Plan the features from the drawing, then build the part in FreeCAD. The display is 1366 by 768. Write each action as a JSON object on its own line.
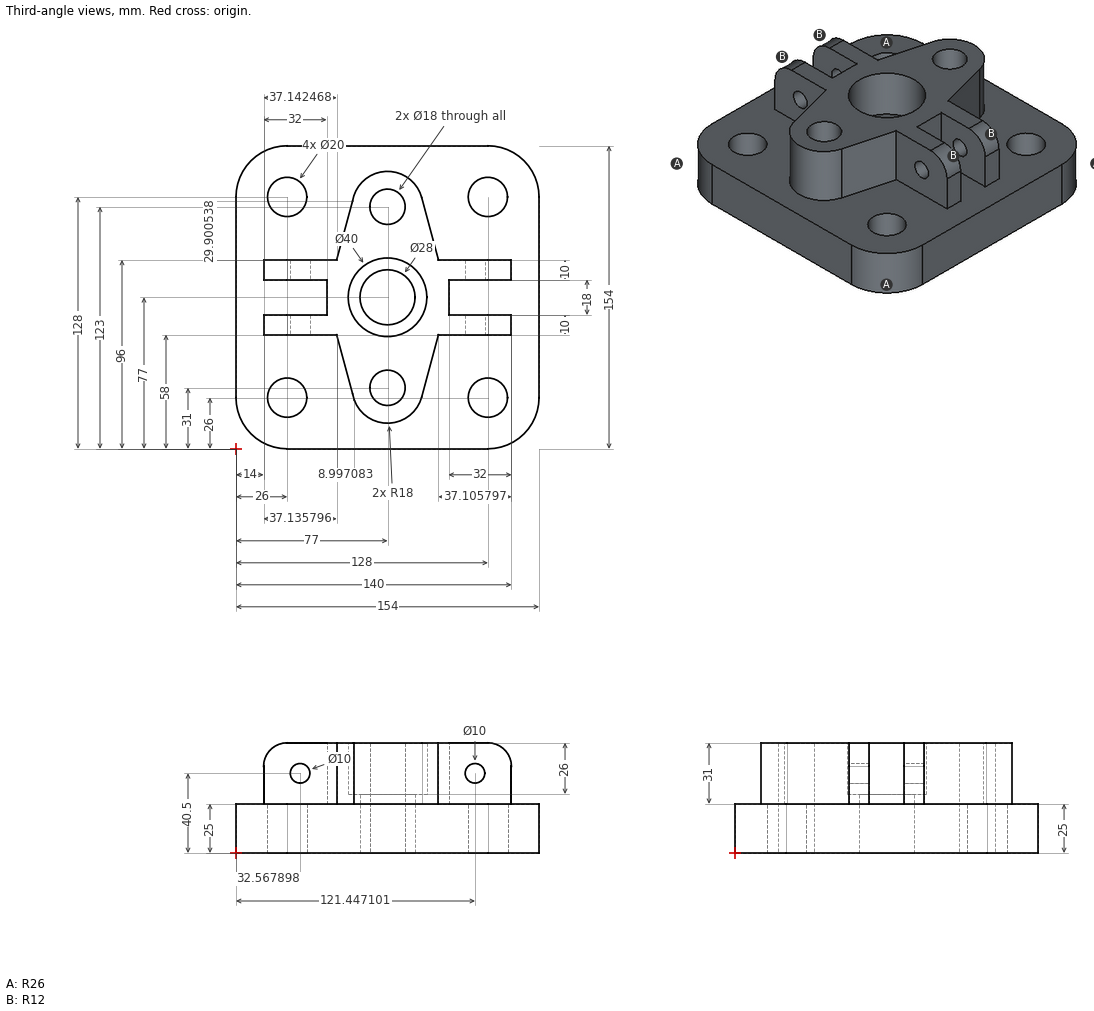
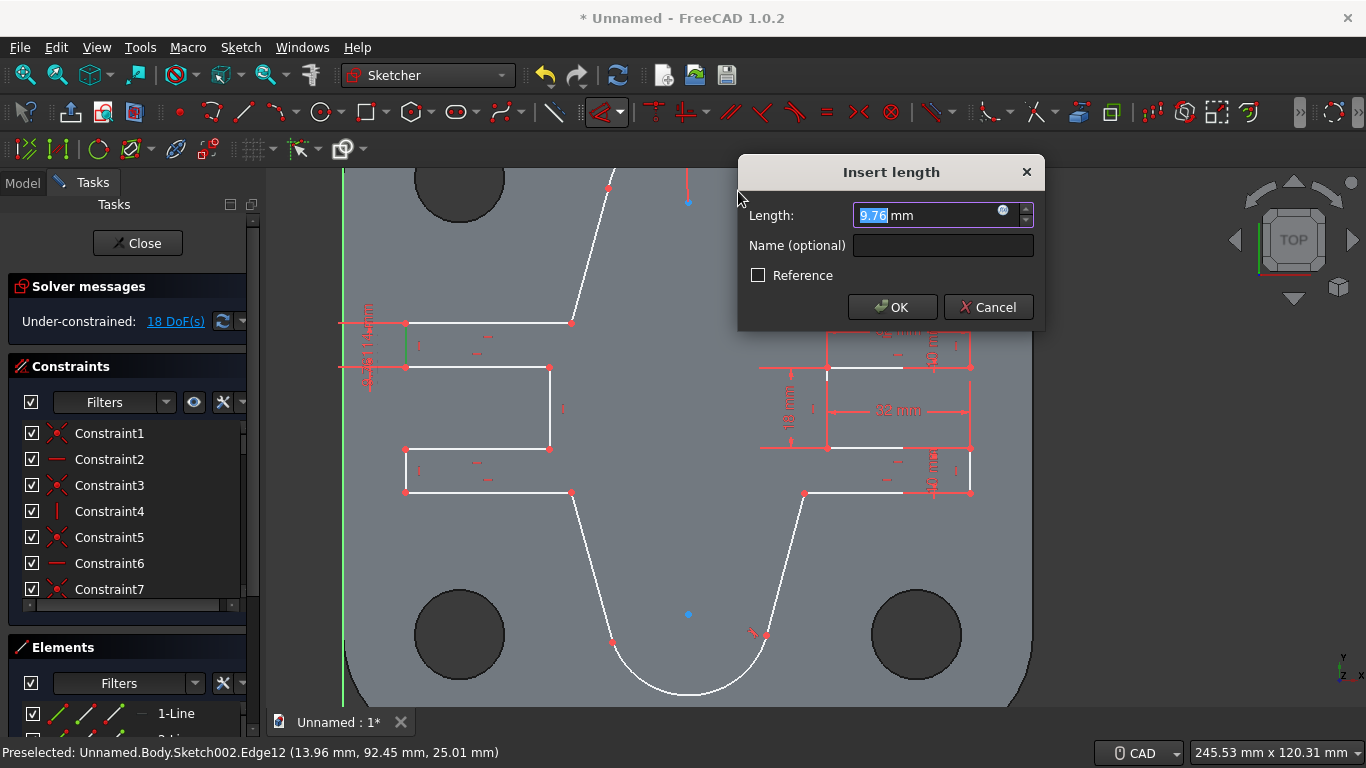
{"action": "type", "text": "10"}
{"action": "key", "text": "Return"}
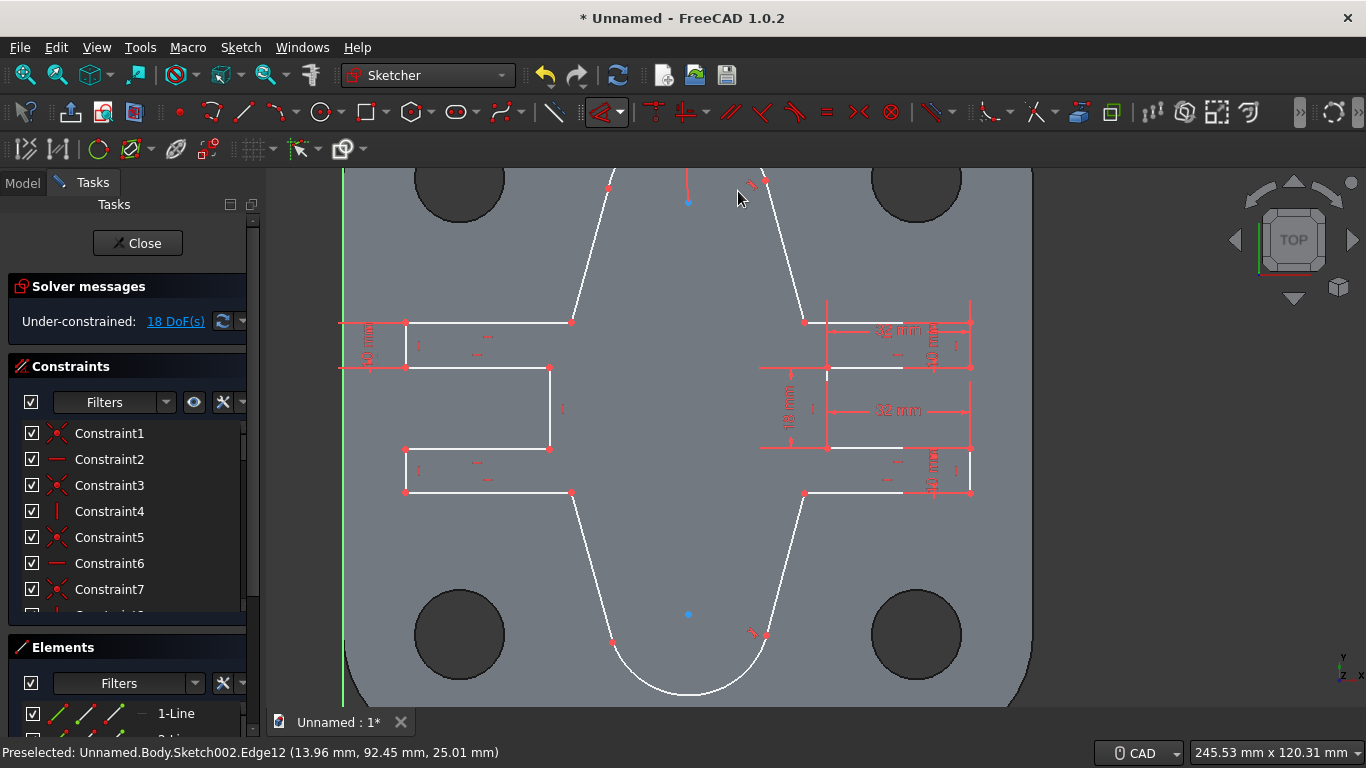
{"action": "left_click", "coordinate": [449, 368]}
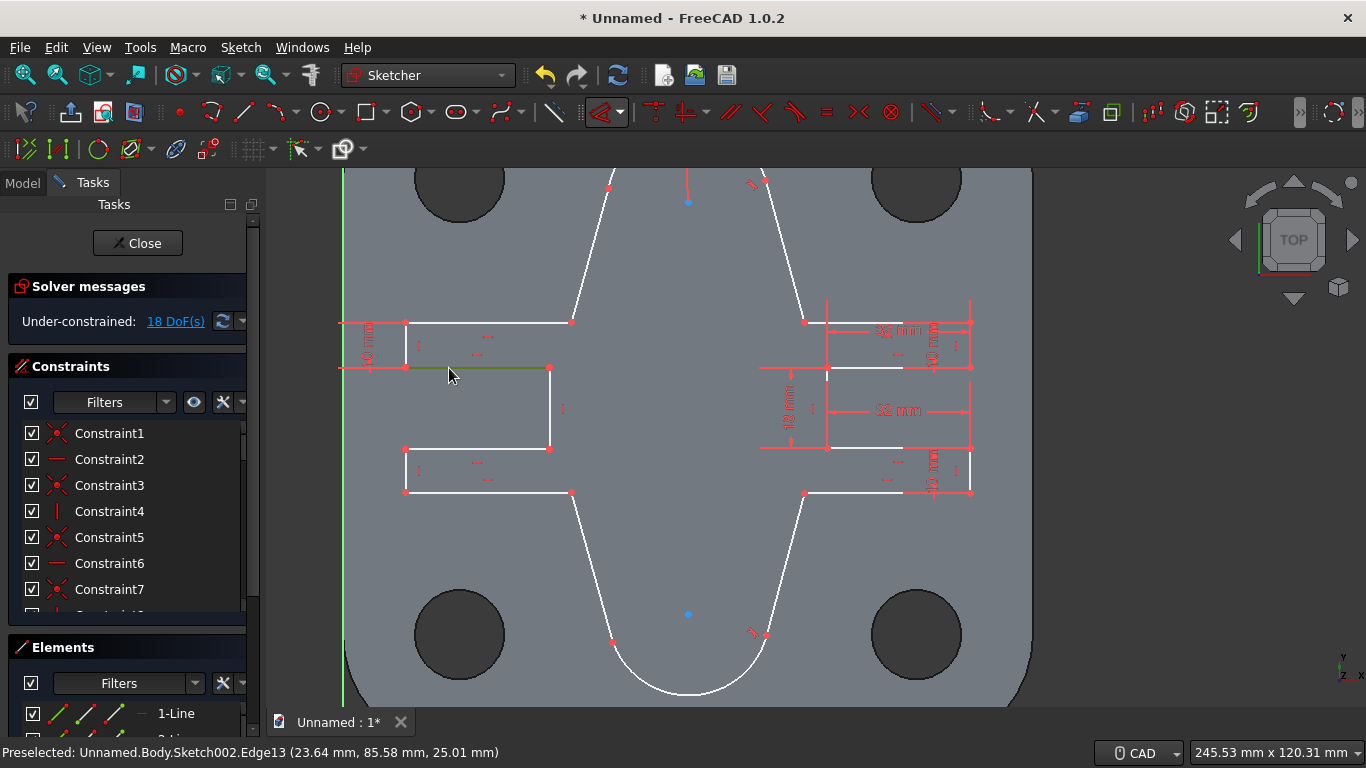
{"action": "left_click", "coordinate": [622, 112]}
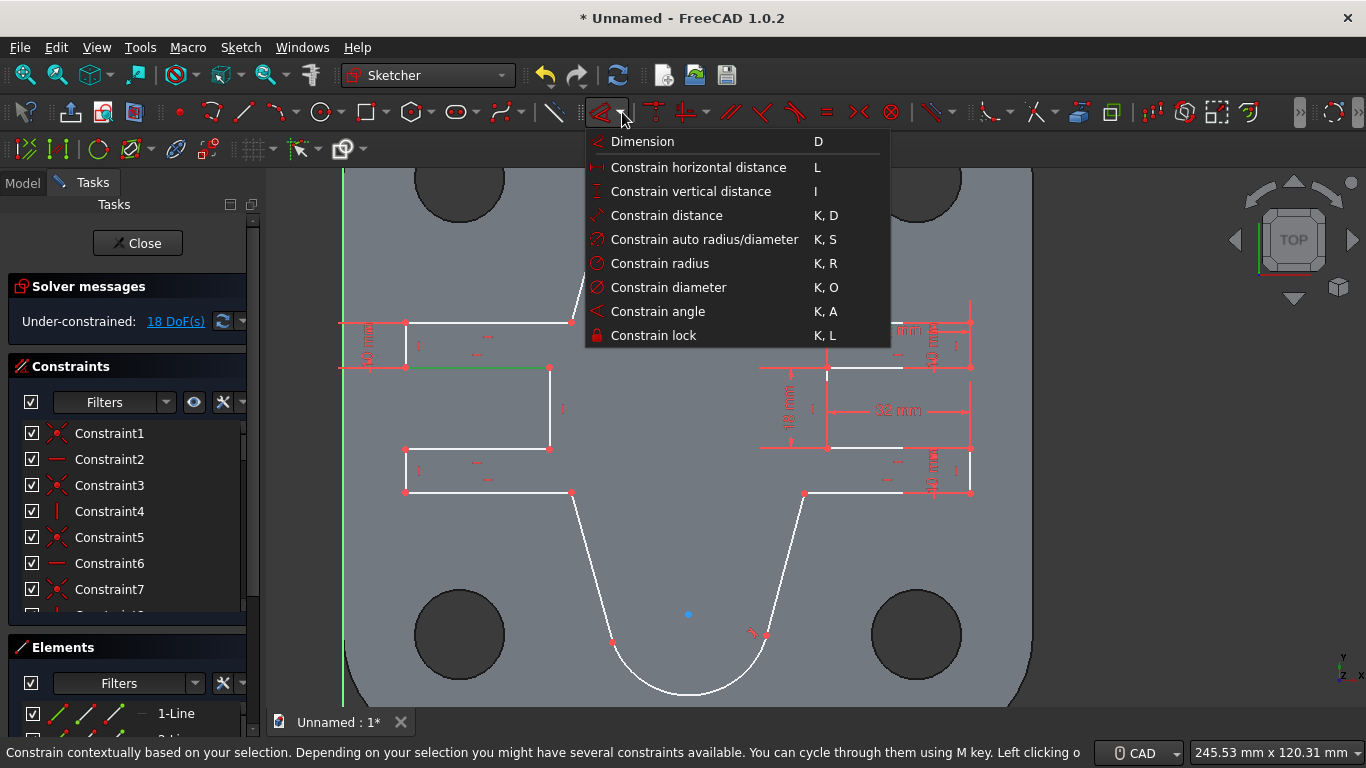
{"action": "left_click", "coordinate": [738, 167]}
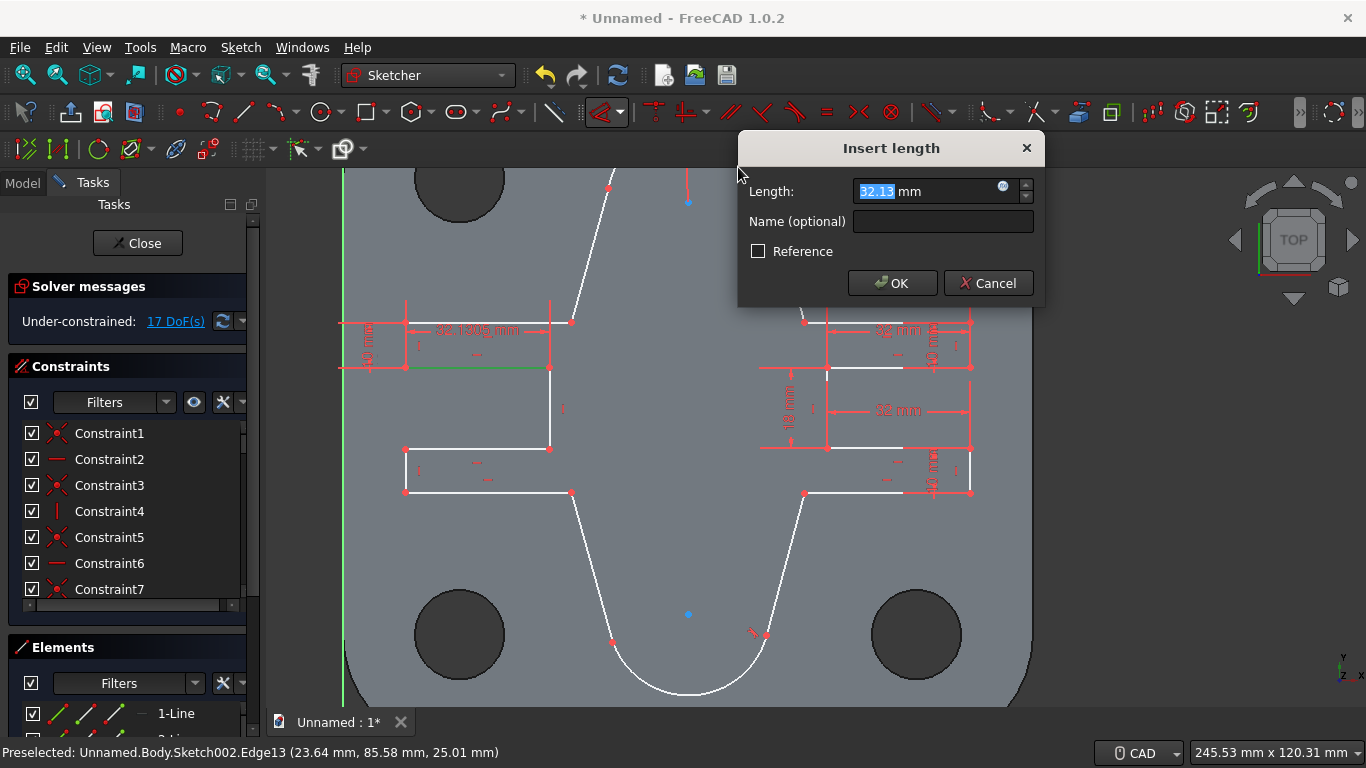
{"action": "type", "text": "32"}
{"action": "key", "text": "Return"}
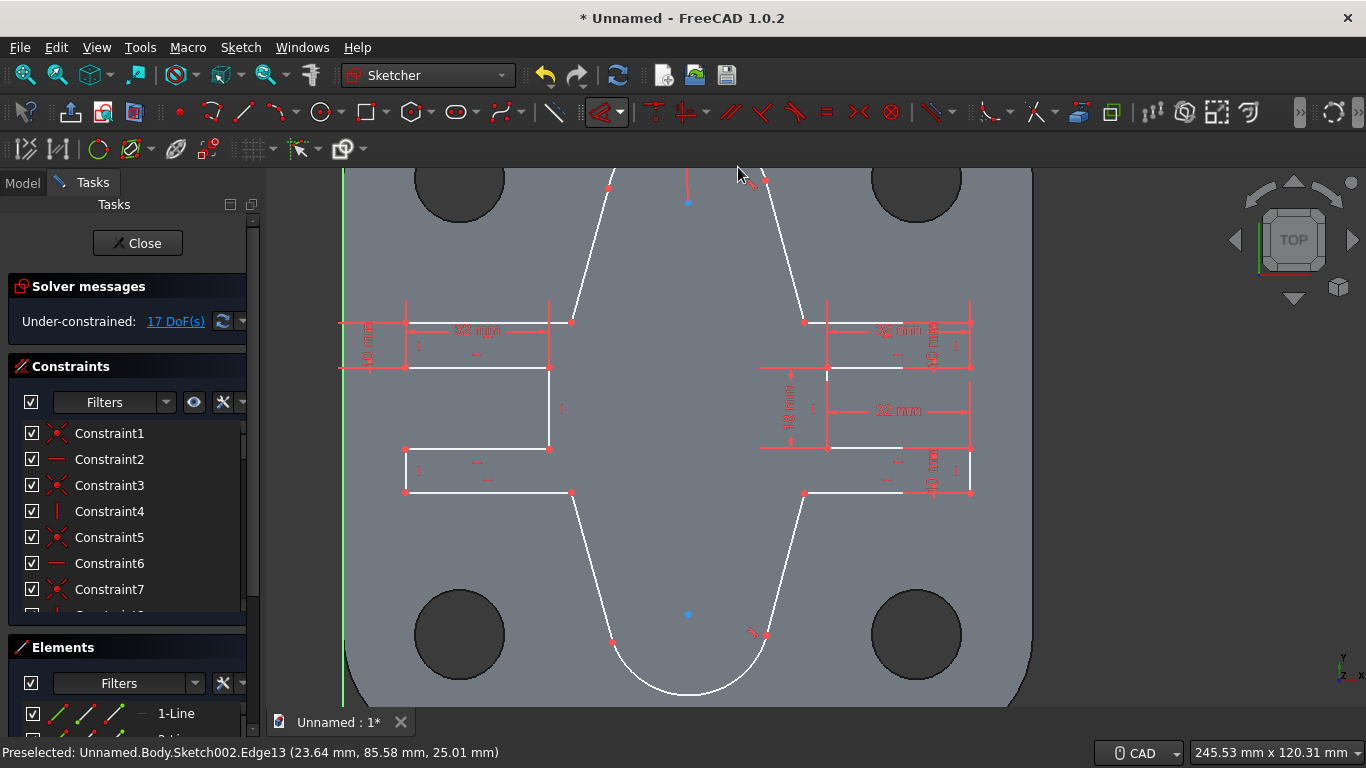
{"action": "left_click", "coordinate": [549, 392]}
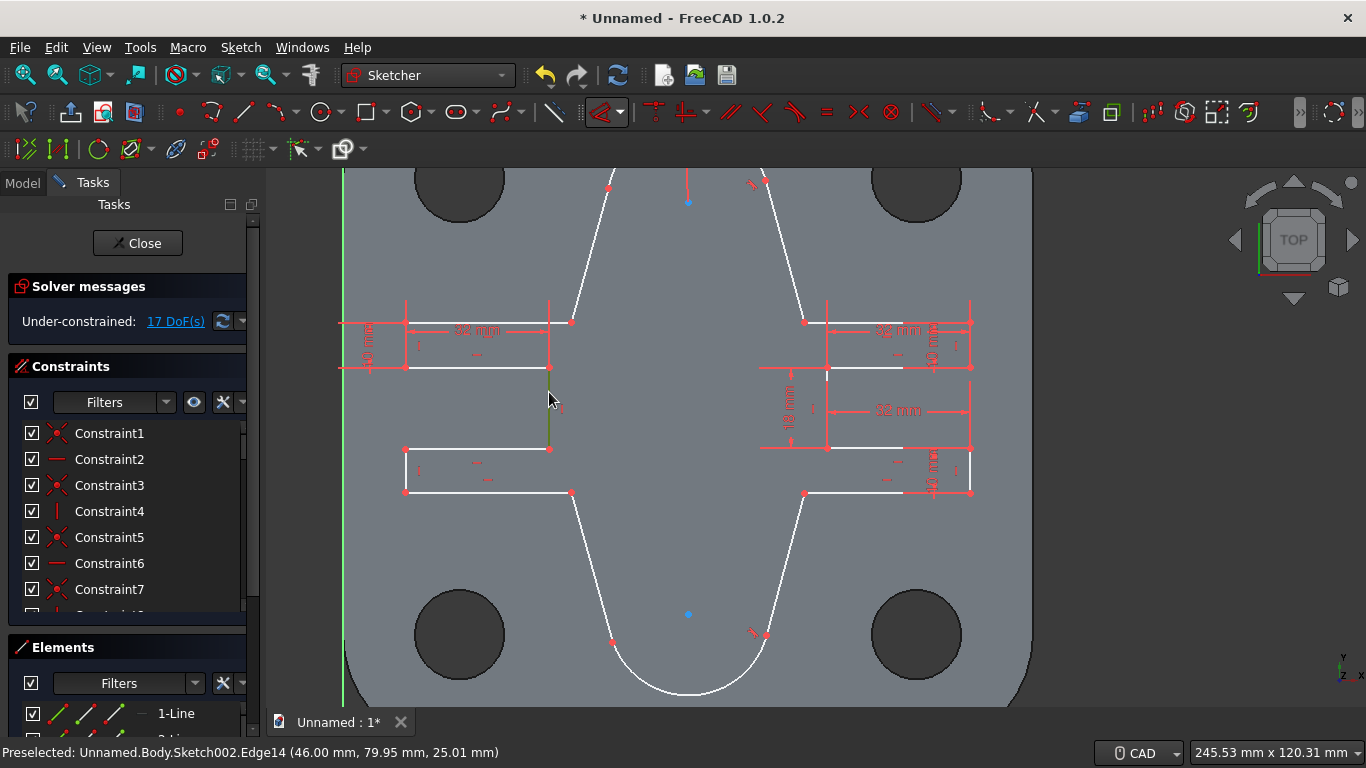
{"action": "left_click", "coordinate": [622, 112]}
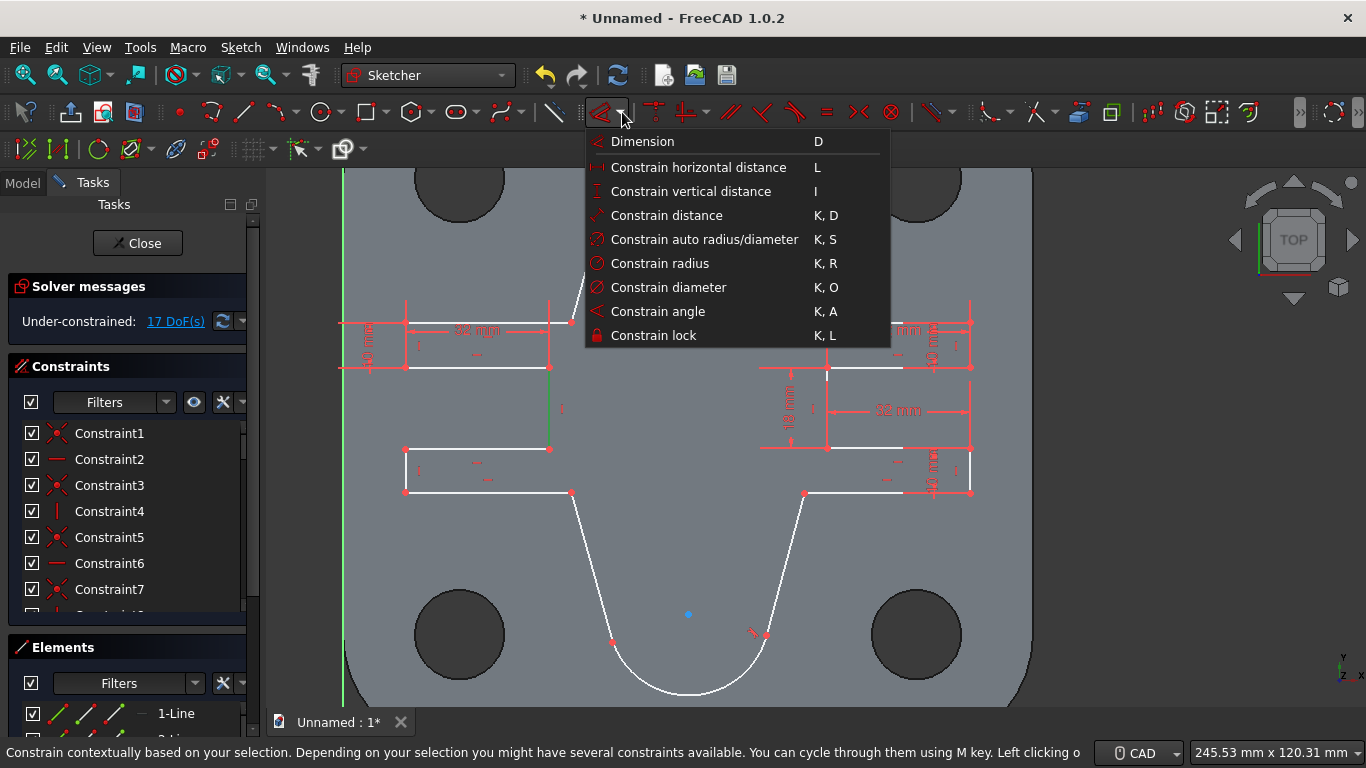
{"action": "left_click", "coordinate": [738, 191]}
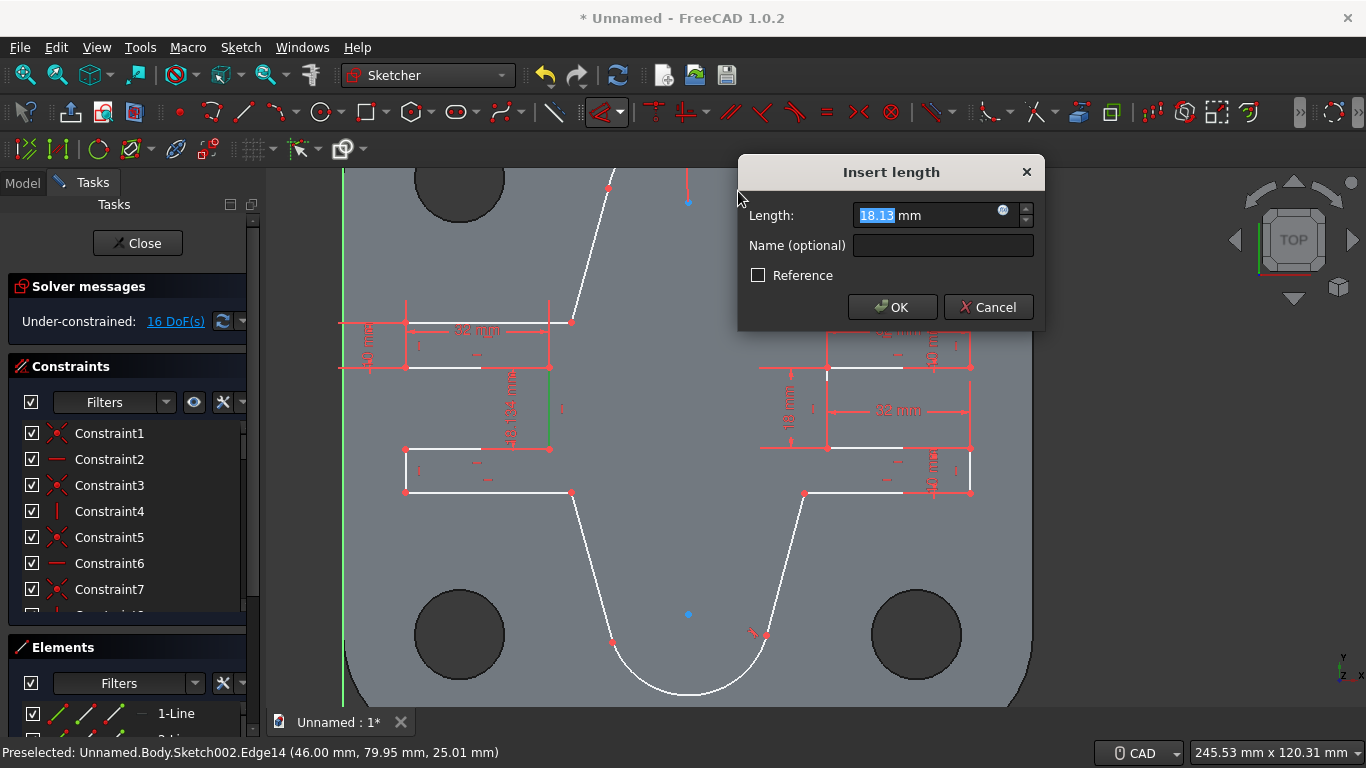
{"action": "type", "text": "18"}
{"action": "key", "text": "Return"}